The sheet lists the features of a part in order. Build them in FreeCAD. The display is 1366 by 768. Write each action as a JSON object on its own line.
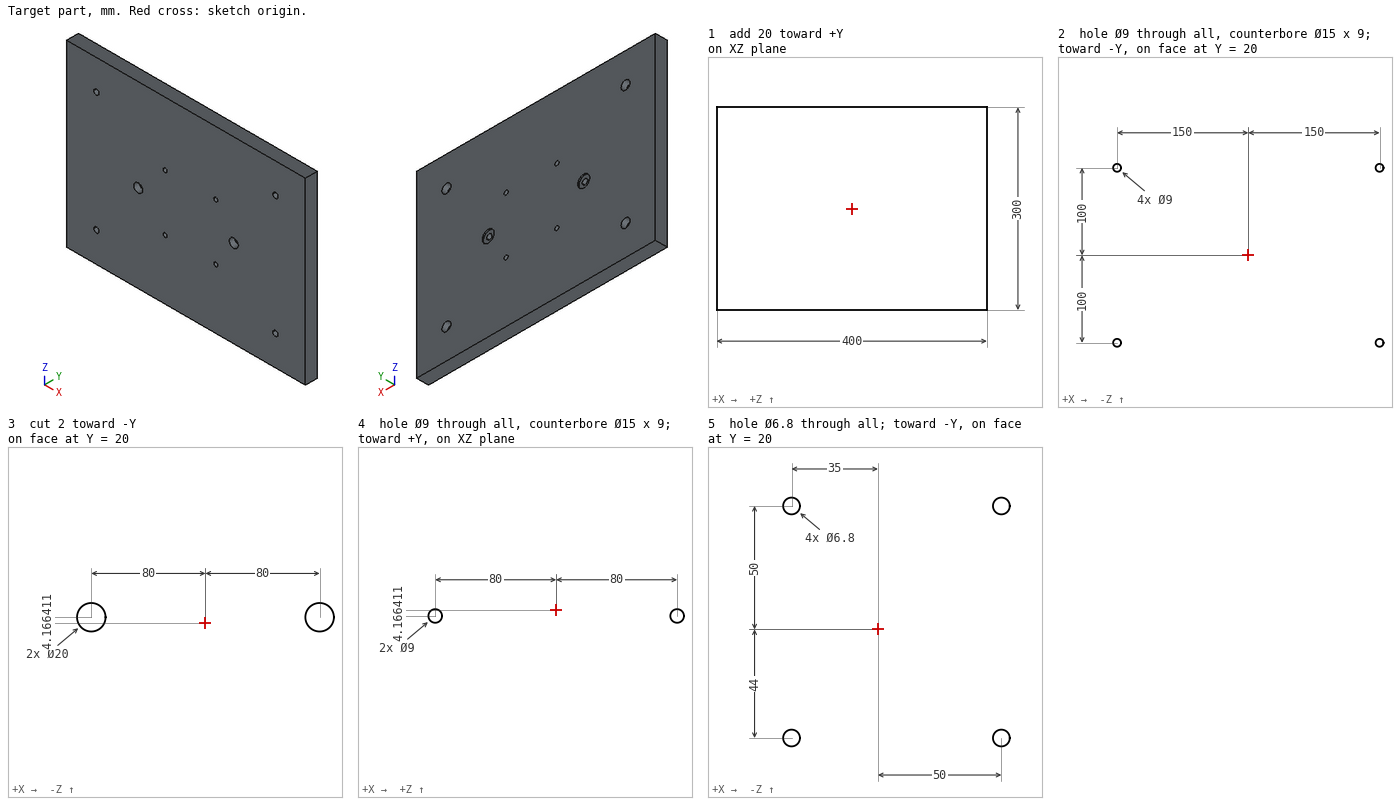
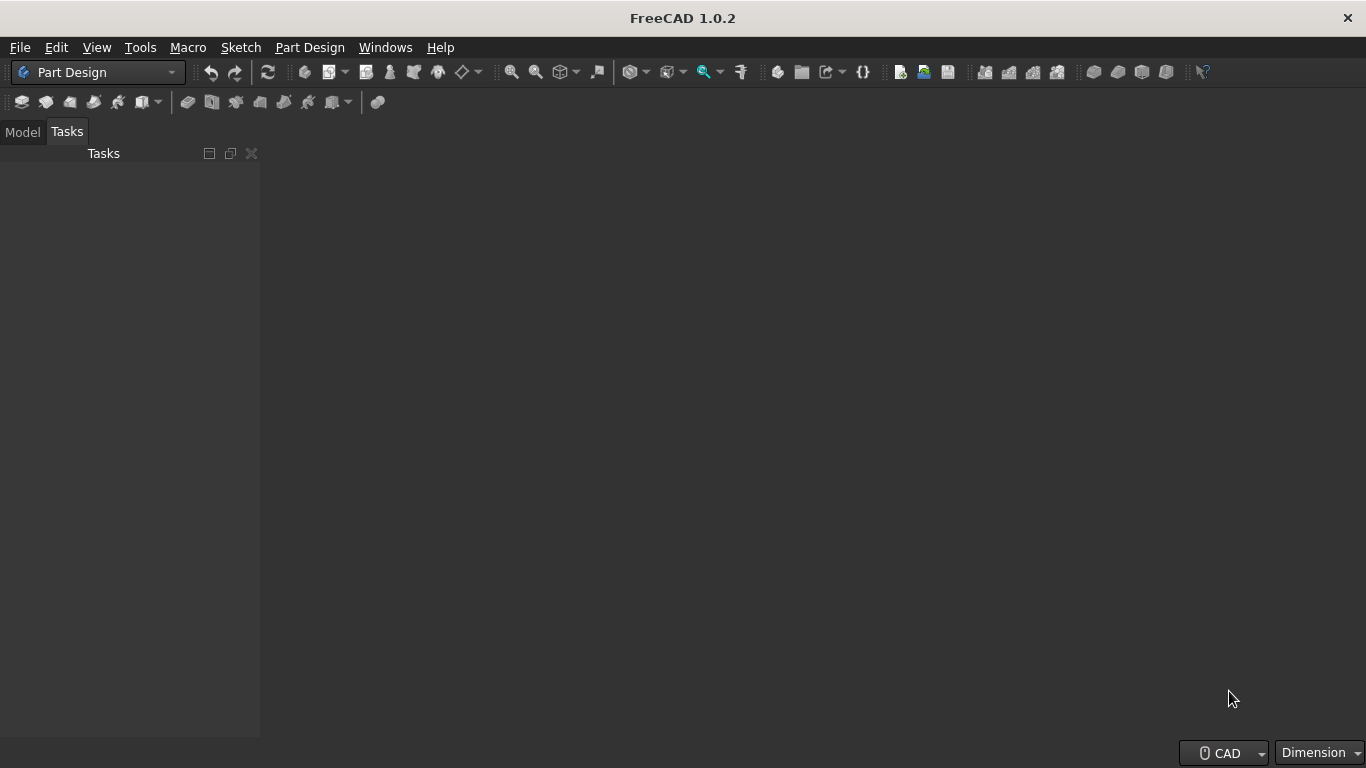
{"action": "left_click", "coordinate": [900, 72]}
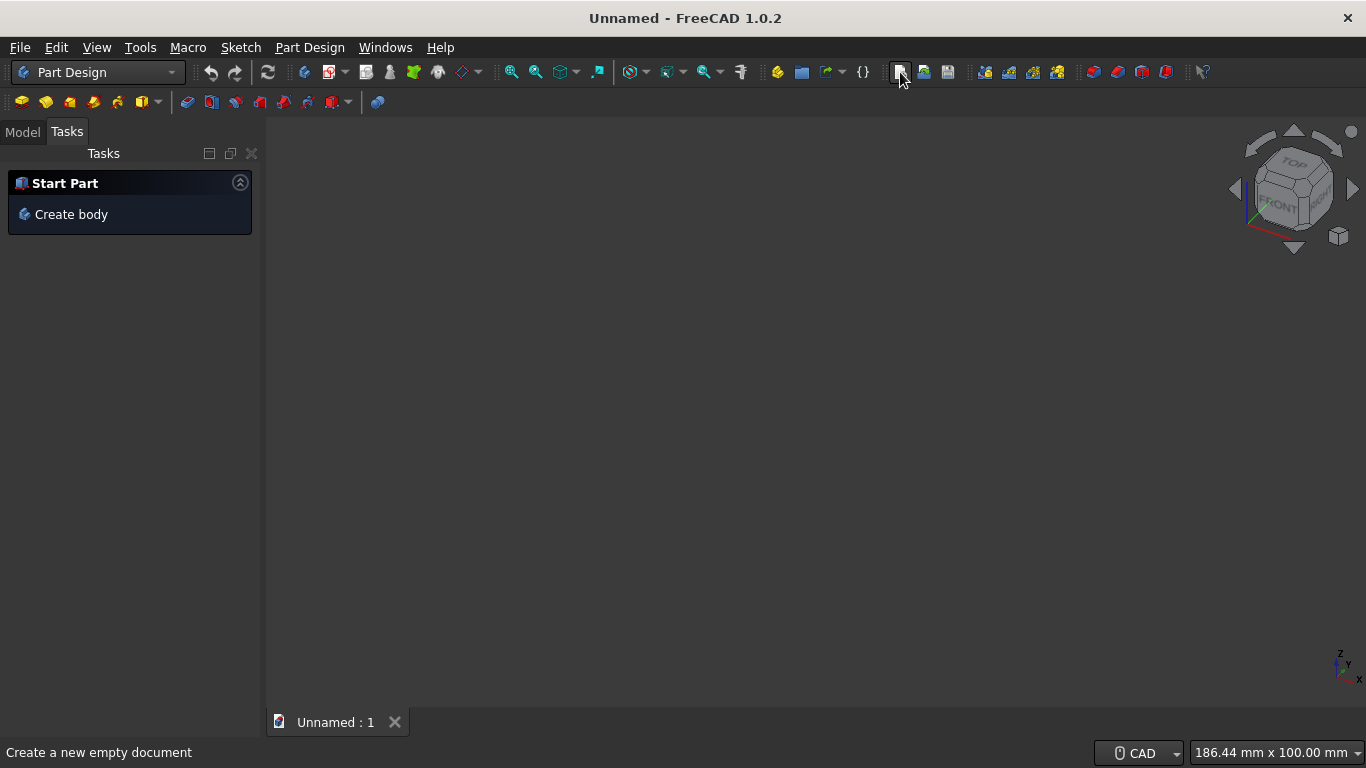
{"action": "left_click", "coordinate": [330, 72]}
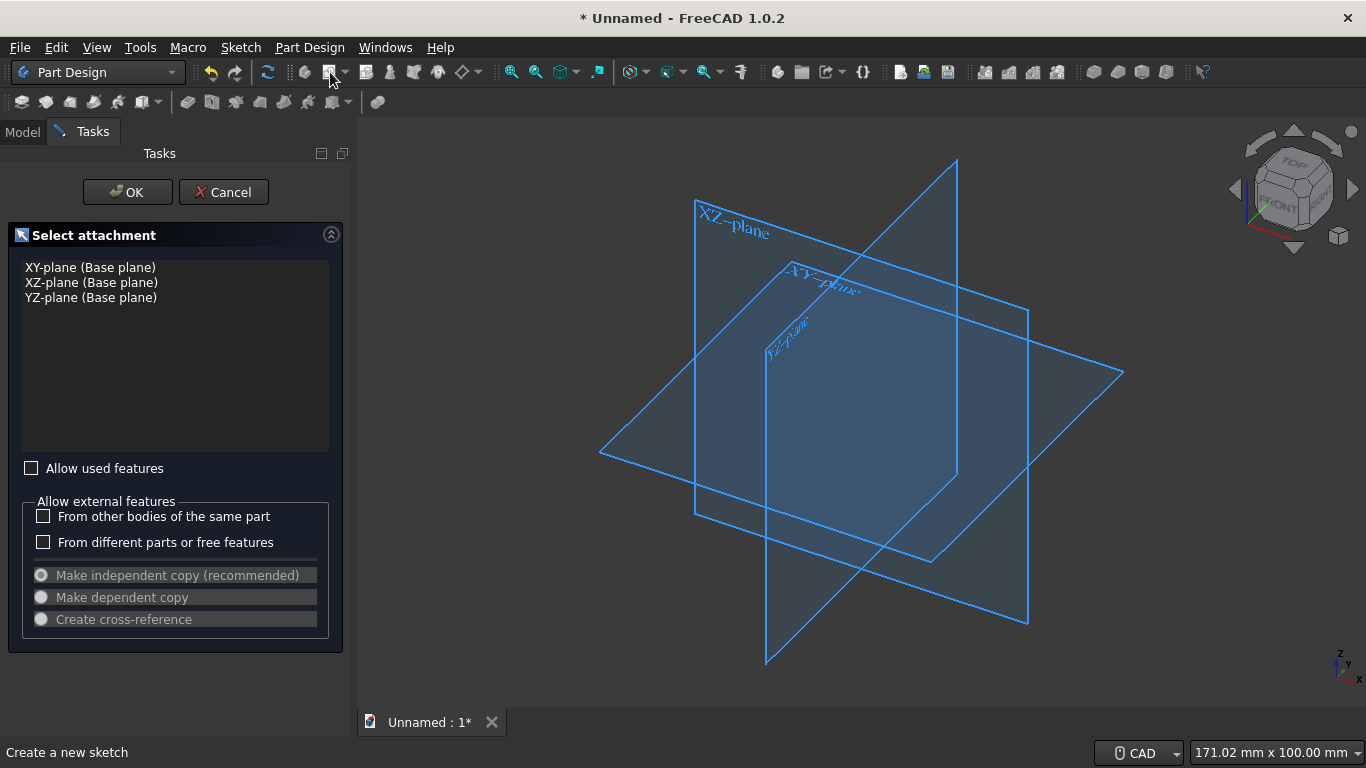
{"action": "left_click", "coordinate": [82, 282]}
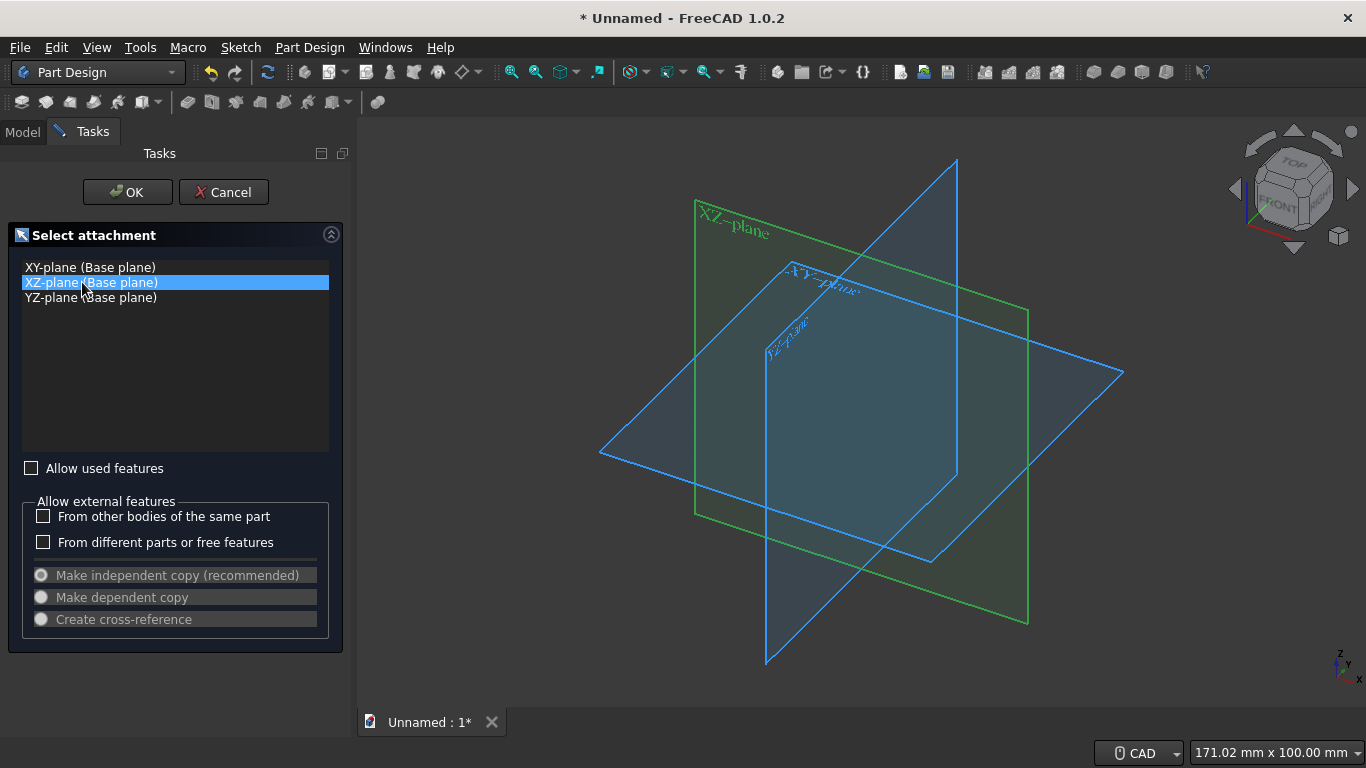
{"action": "left_click", "coordinate": [128, 192]}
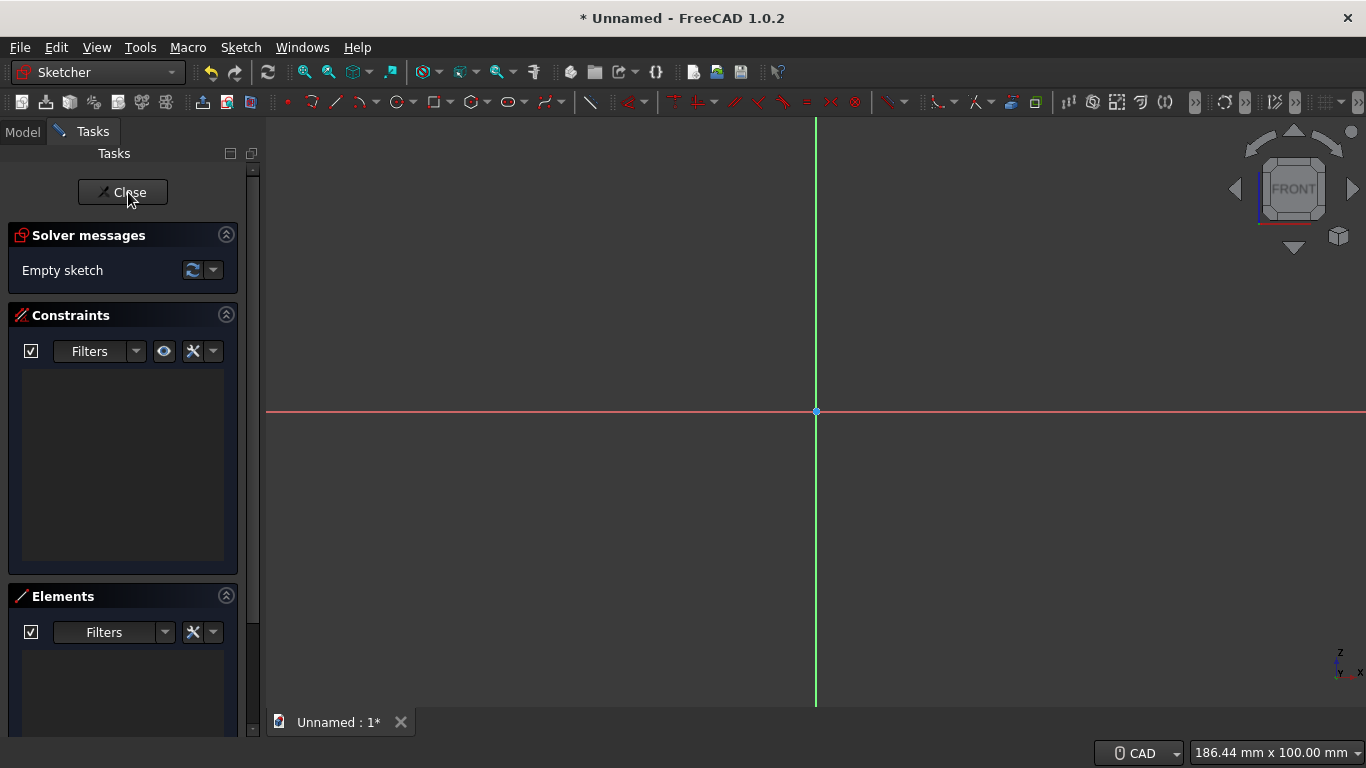
{"action": "scroll", "coordinate": [730, 412], "scroll_direction": "down", "scroll_amount": 8}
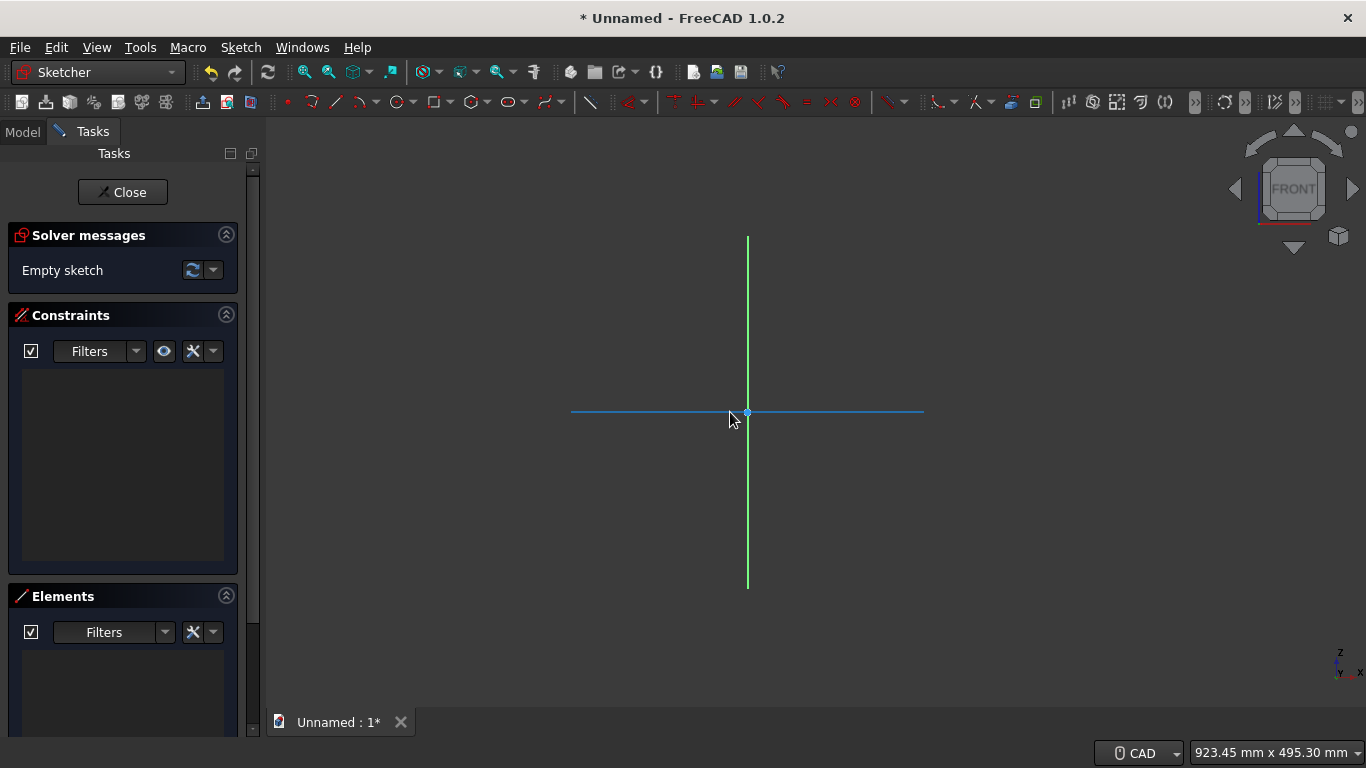
{"action": "key", "text": "g v"}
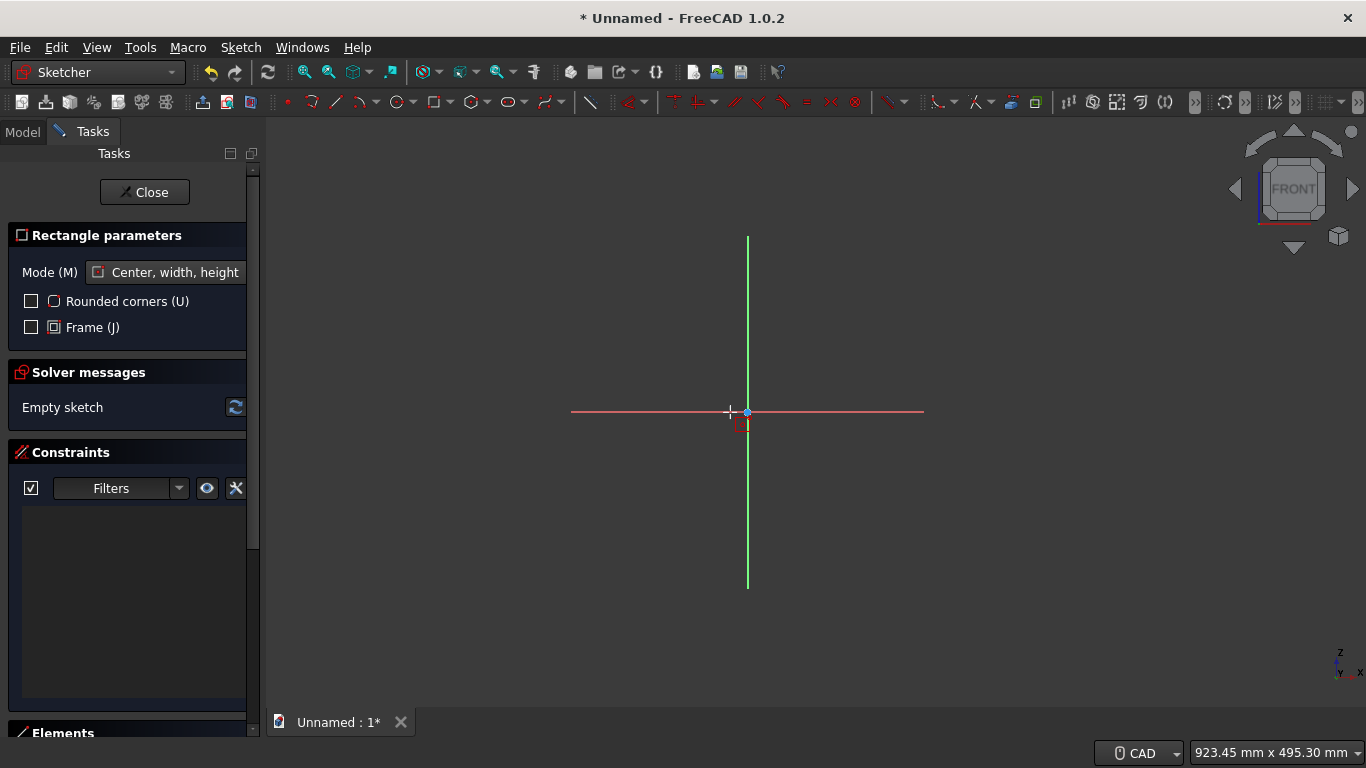
{"action": "left_click", "coordinate": [748, 412]}
{"action": "left_click", "coordinate": [986, 234]}
{"action": "key", "text": "Escape"}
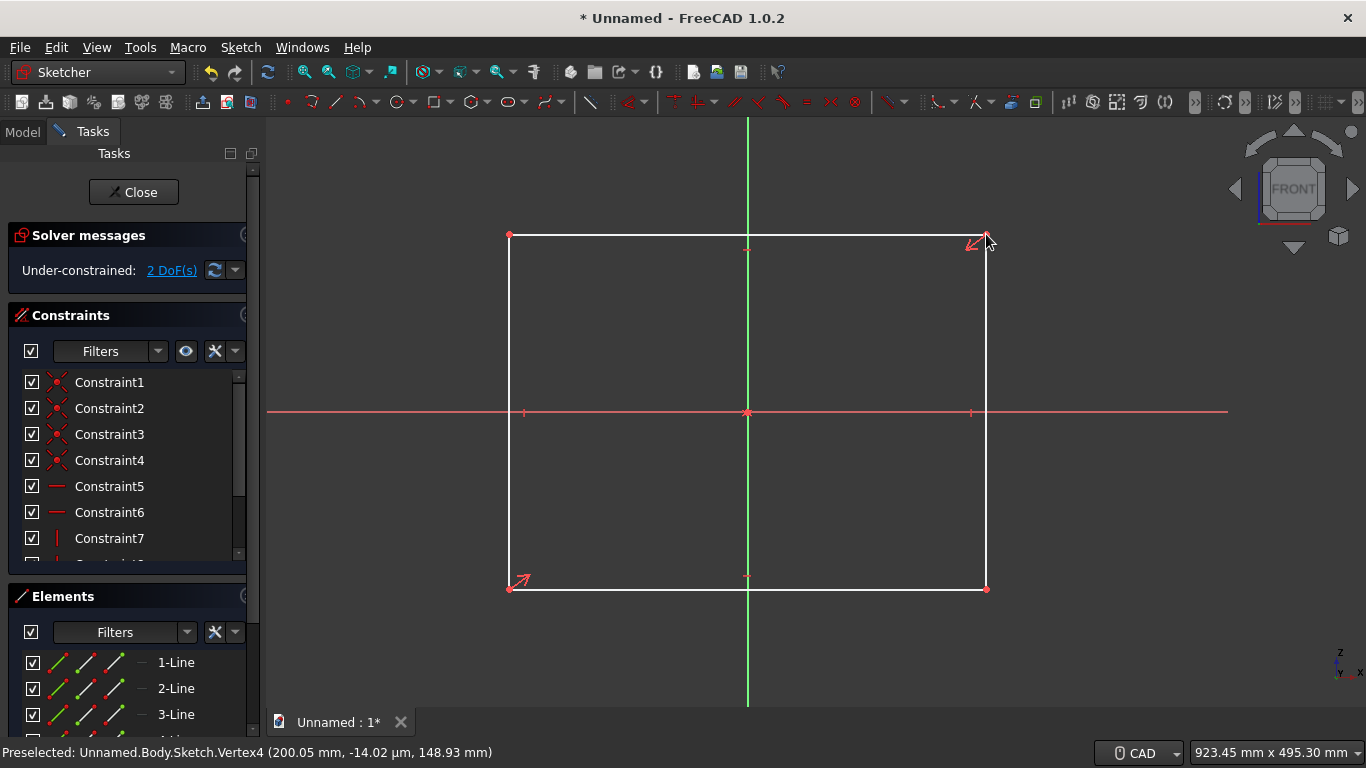
{"action": "left_click", "coordinate": [628, 102]}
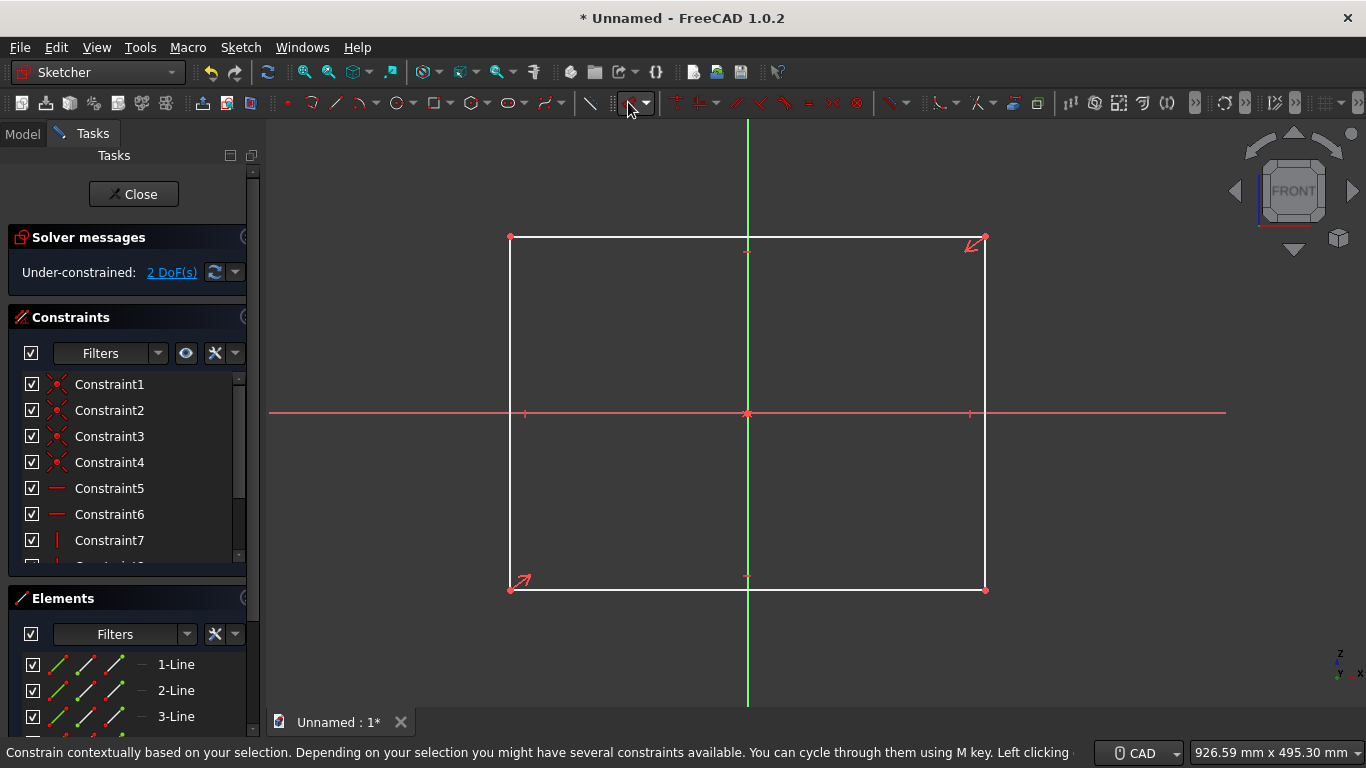
{"action": "left_click", "coordinate": [653, 590]}
{"action": "left_click", "coordinate": [639, 624]}